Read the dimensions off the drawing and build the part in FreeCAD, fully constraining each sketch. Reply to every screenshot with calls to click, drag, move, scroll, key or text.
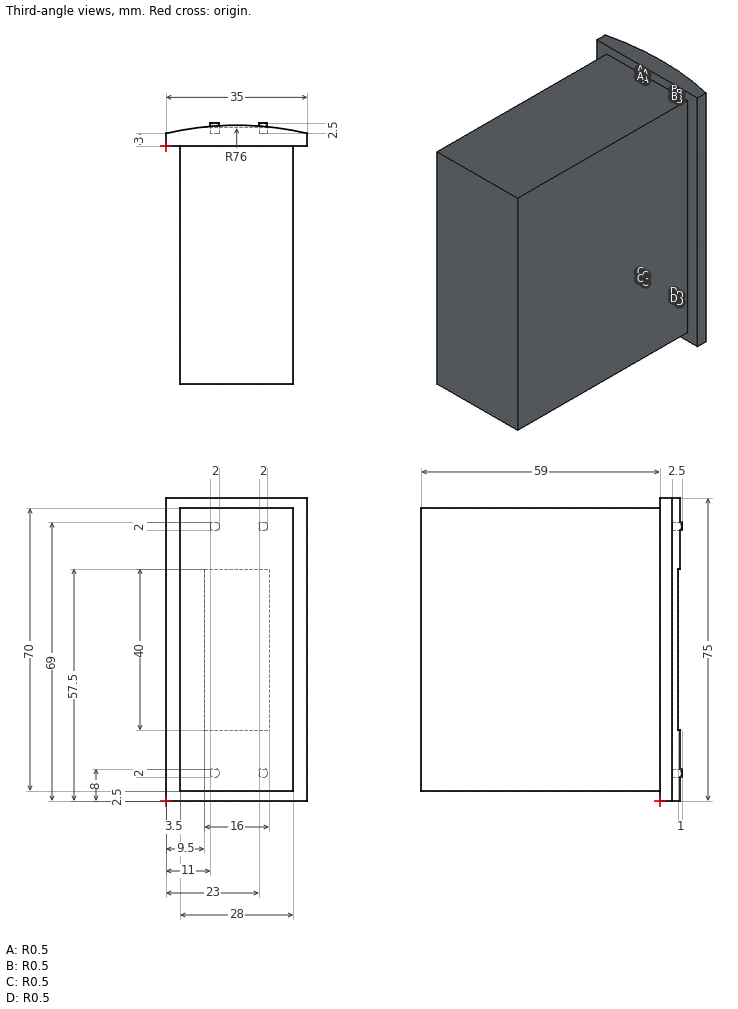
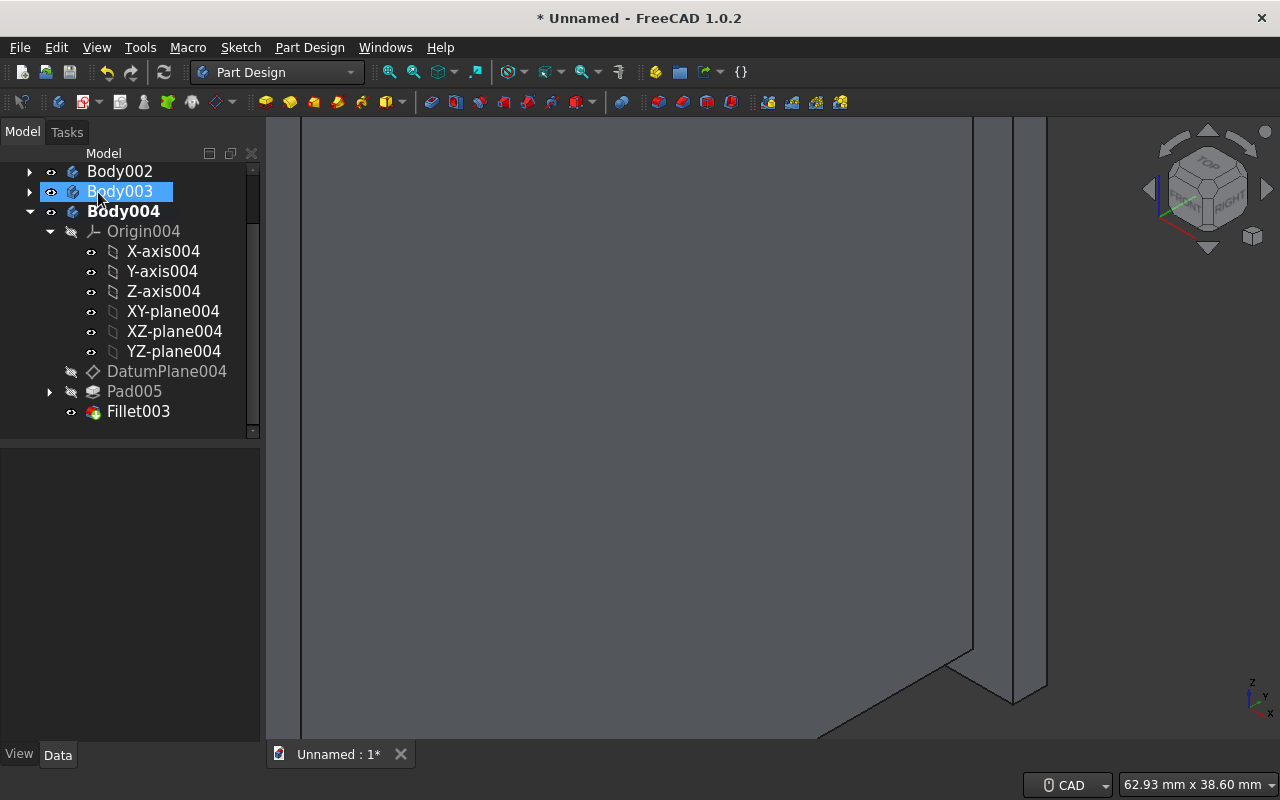
key(v)
key(f)